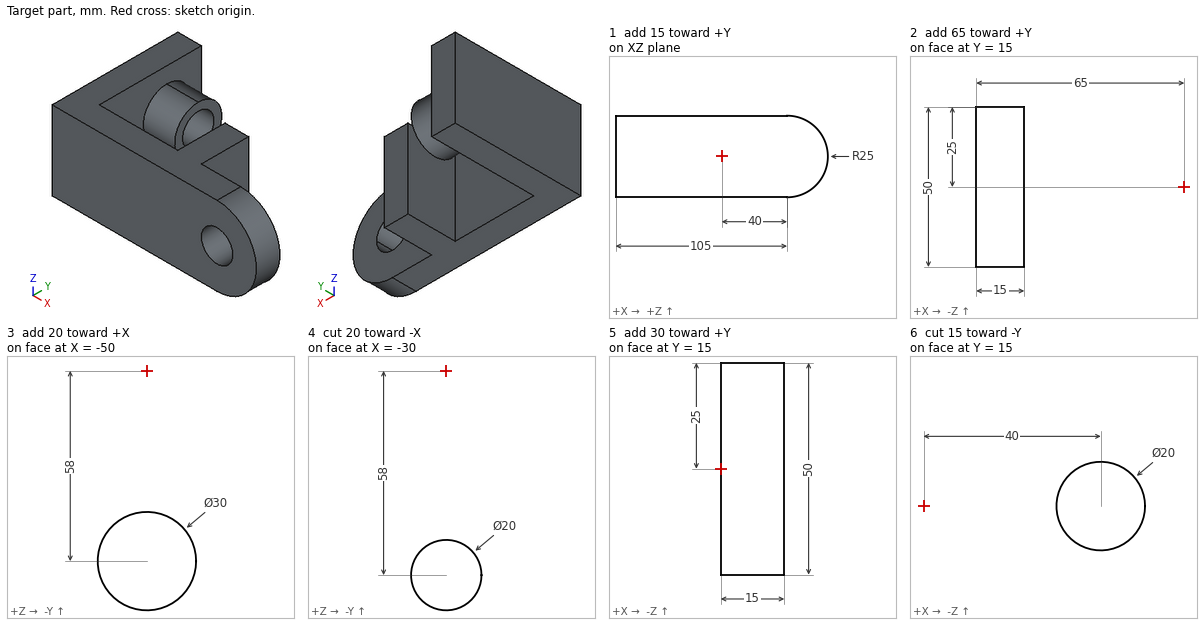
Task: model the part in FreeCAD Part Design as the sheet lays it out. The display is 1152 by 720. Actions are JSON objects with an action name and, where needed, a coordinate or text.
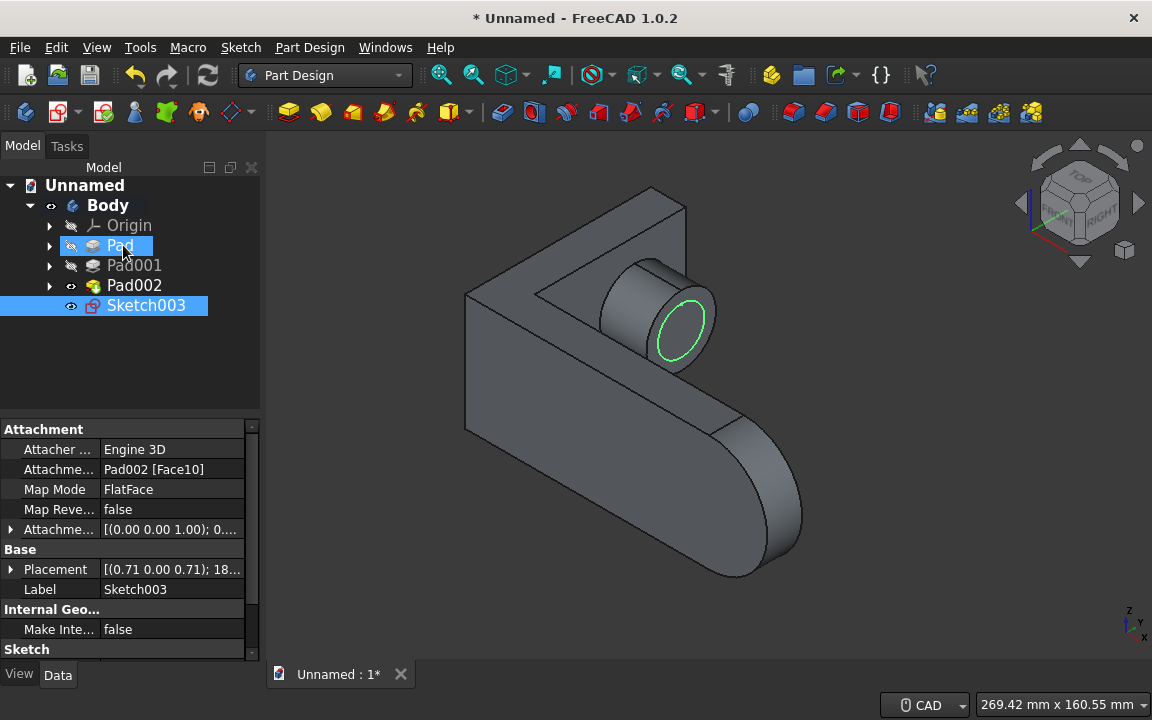
{"action": "left_click", "coordinate": [504, 112]}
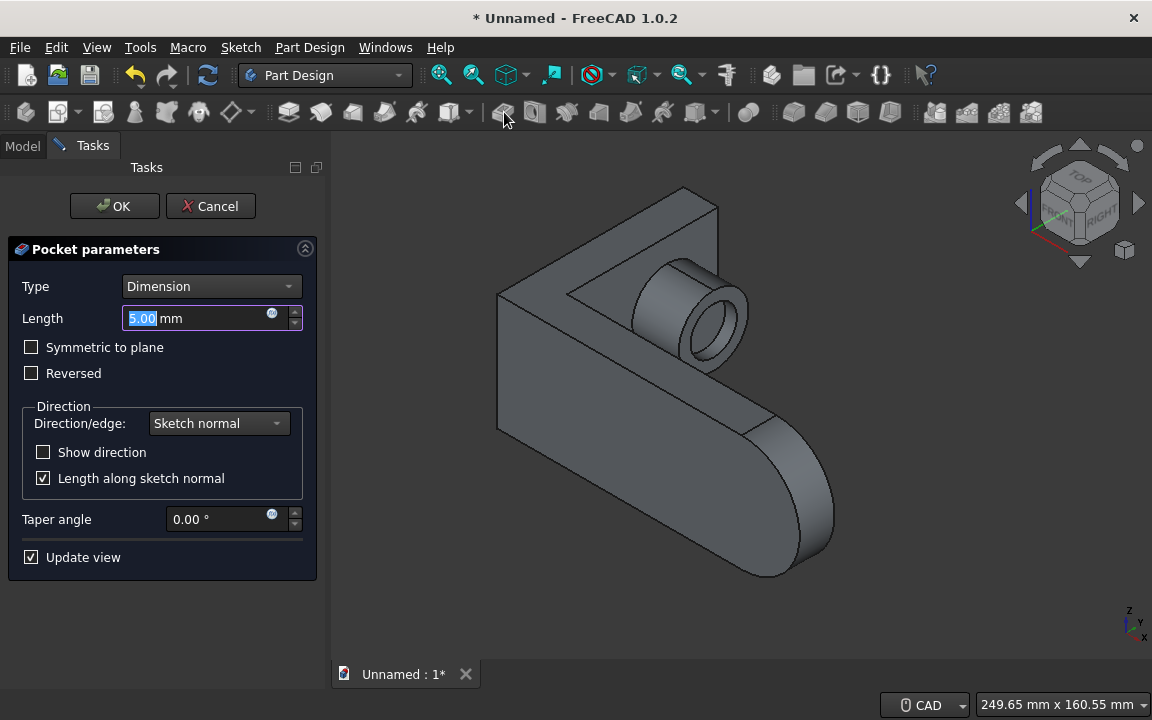
{"action": "type", "text": "20"}
{"action": "key", "text": "Tab"}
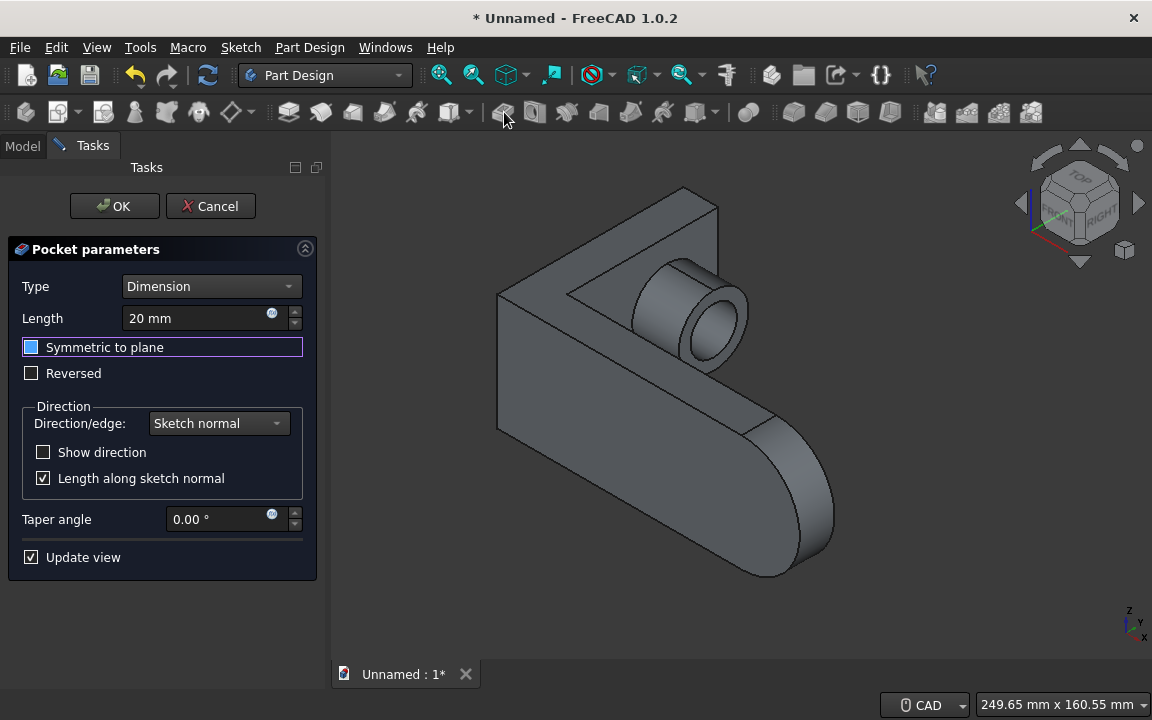
{"action": "left_click", "coordinate": [115, 206]}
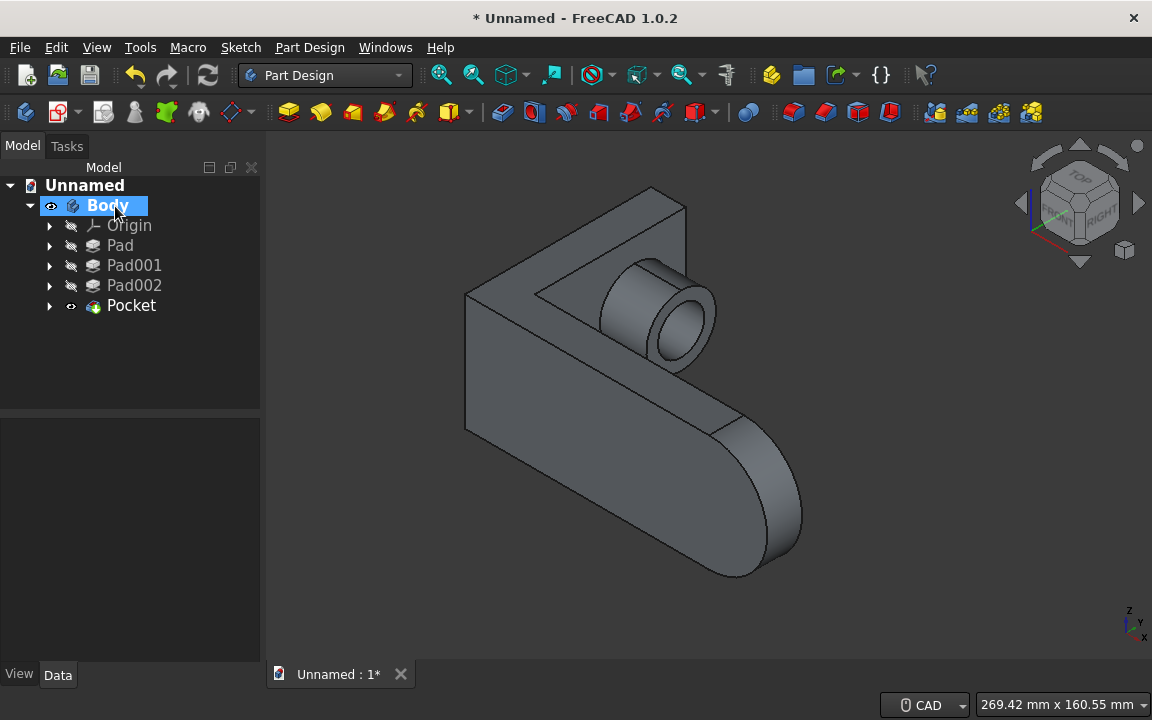
{"action": "key", "text": "4"}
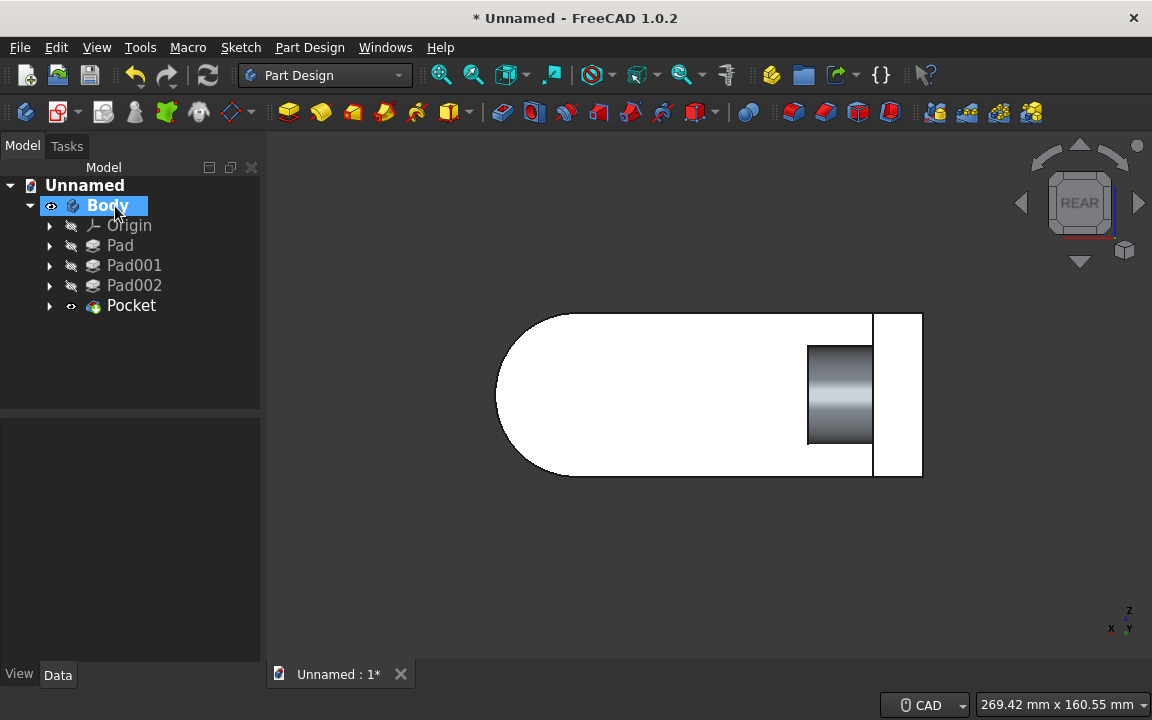
{"action": "left_click", "coordinate": [630, 394]}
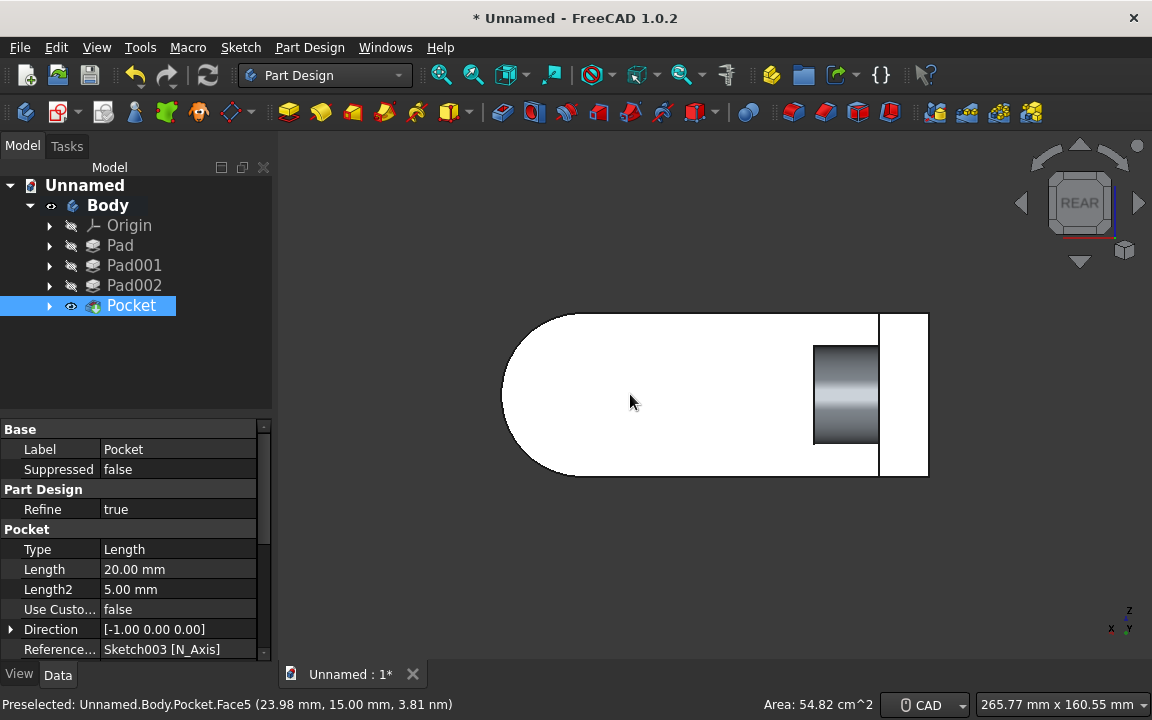
{"action": "left_click", "coordinate": [58, 112]}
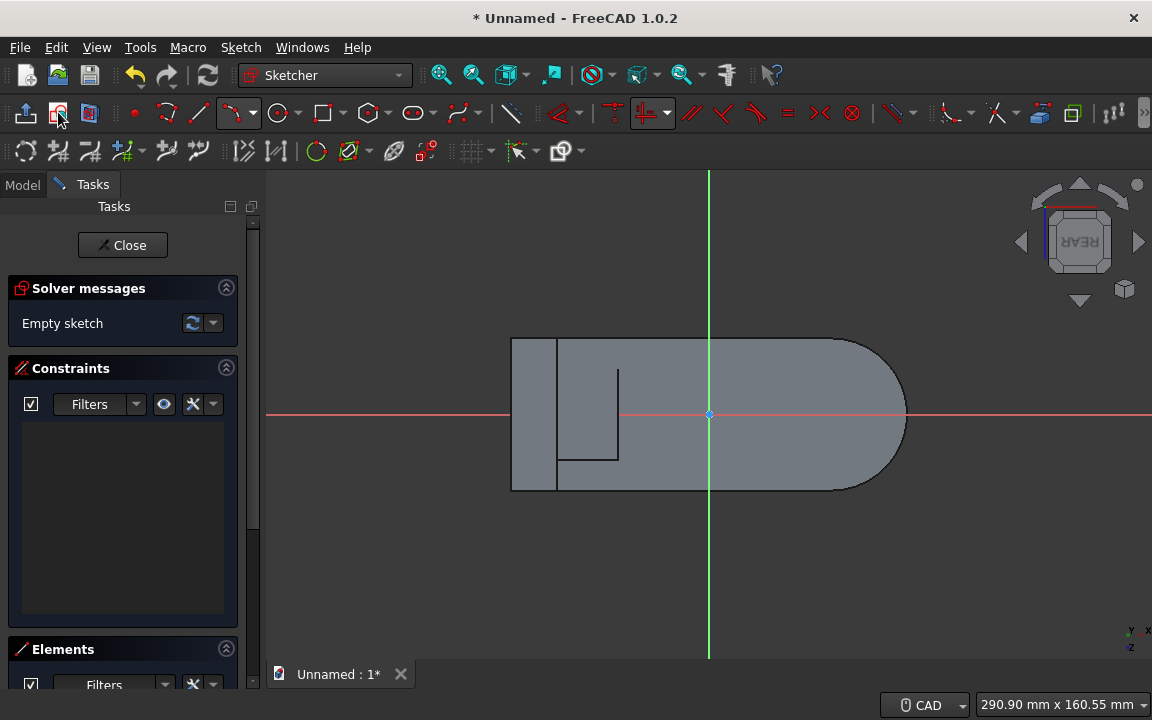
{"action": "scroll", "coordinate": [843, 415], "scroll_direction": "up", "scroll_amount": 3}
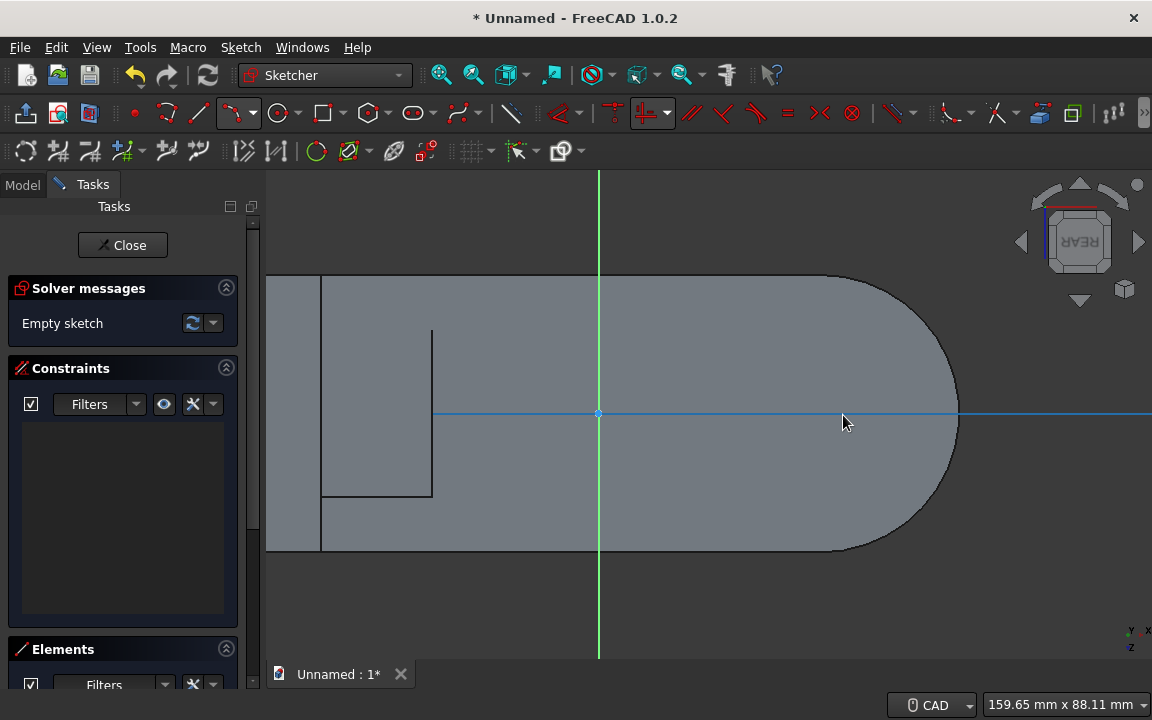
{"action": "left_click", "coordinate": [324, 114]}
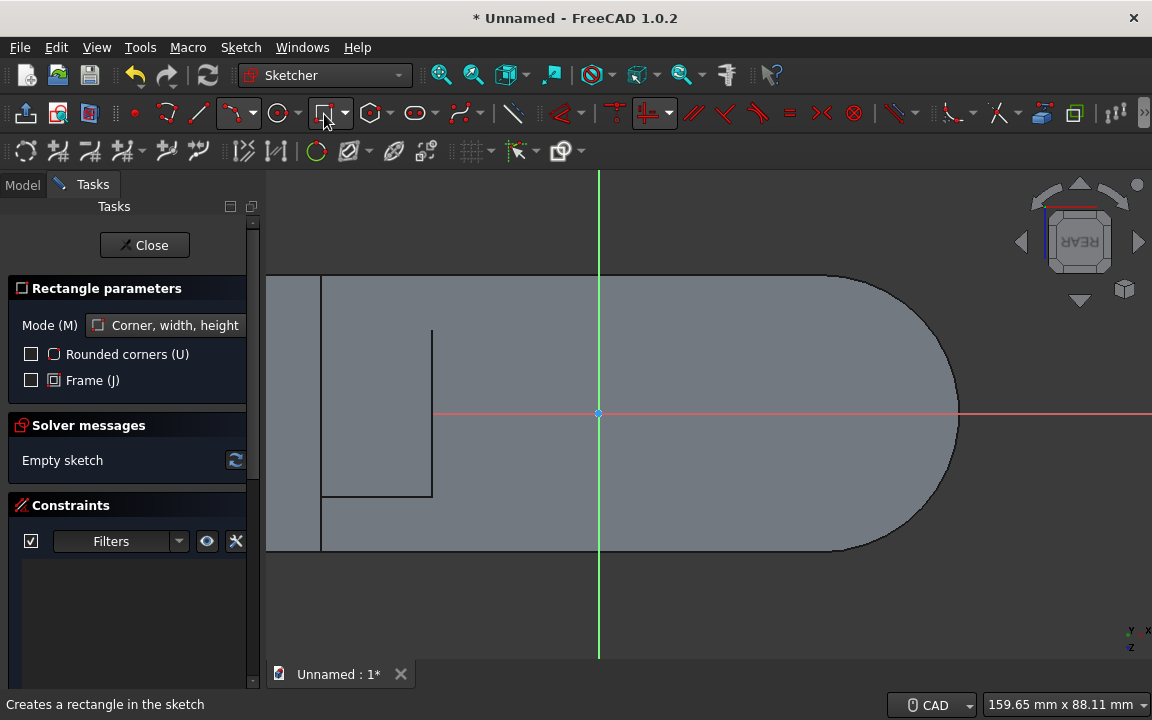
{"action": "left_click", "coordinate": [599, 275]}
{"action": "mouse_move", "coordinate": [682, 552]}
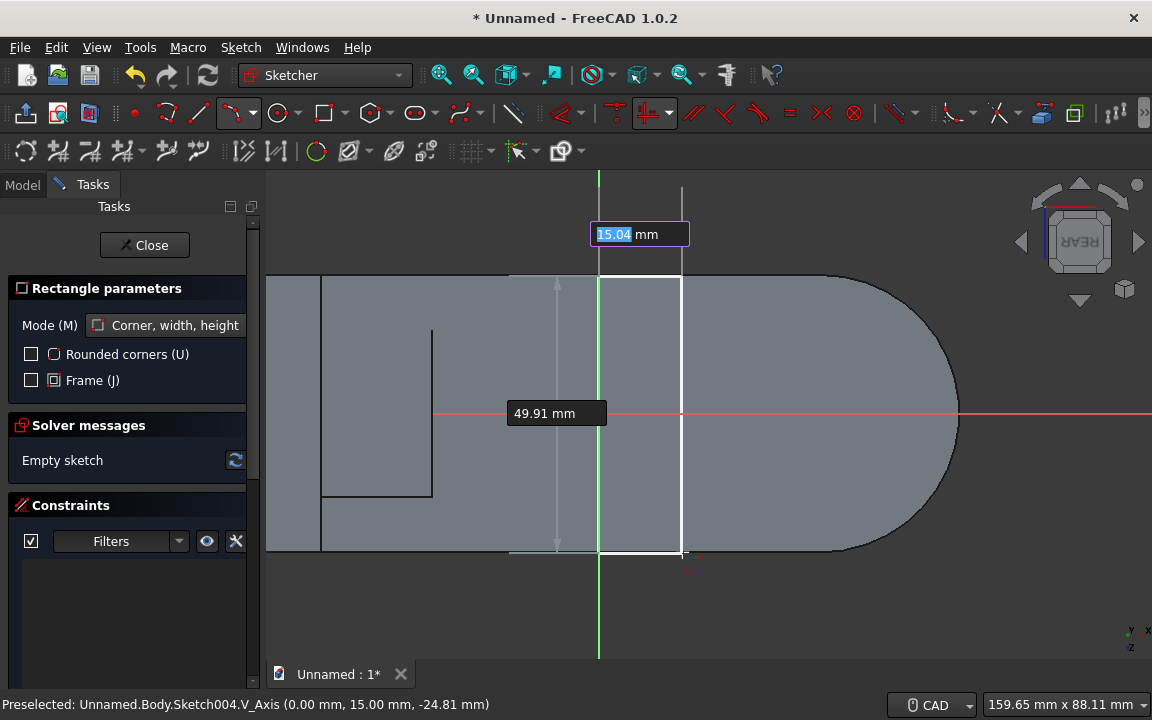
{"action": "type", "text": "15"}
{"action": "key", "text": "Tab"}
{"action": "type", "text": "50"}
{"action": "key", "text": "Return"}
{"action": "key", "text": "Escape"}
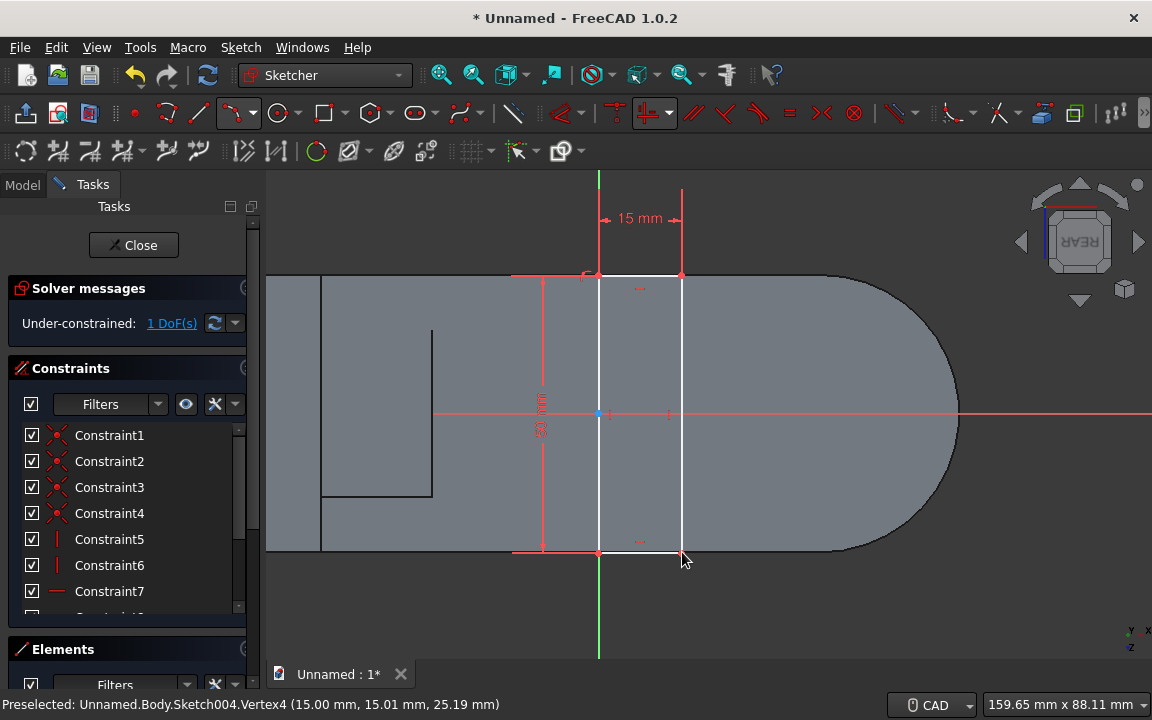
{"action": "left_click", "coordinate": [560, 114]}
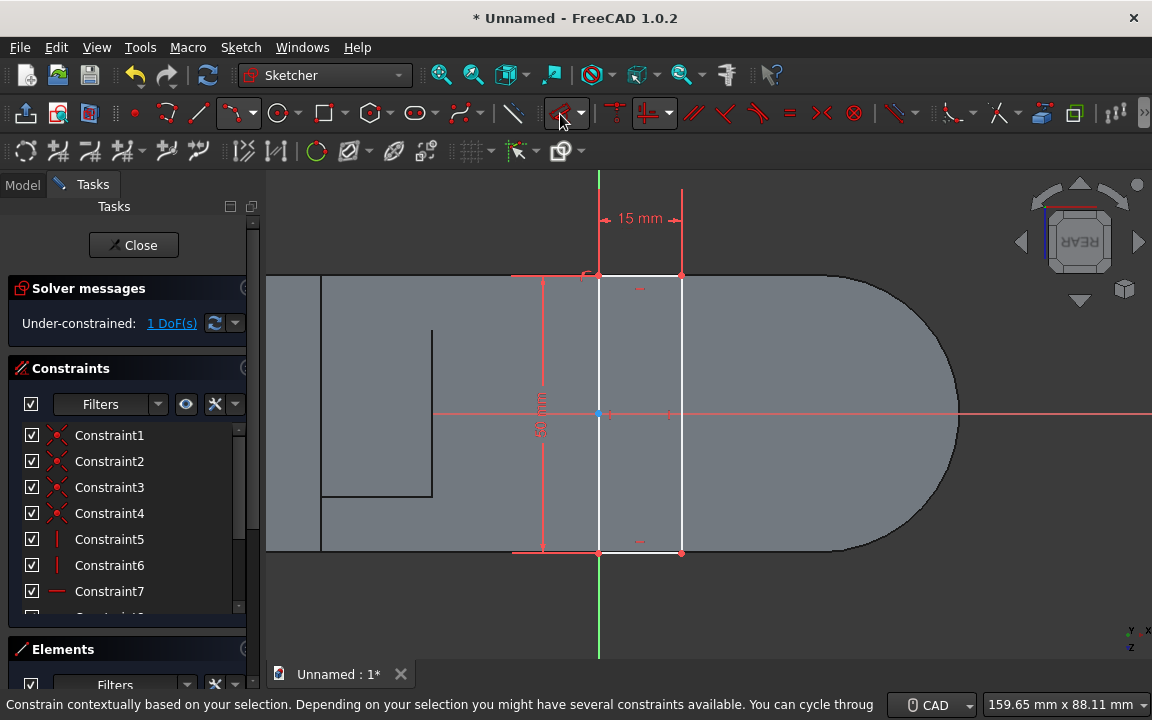
{"action": "left_click", "coordinate": [599, 276]}
{"action": "left_click", "coordinate": [565, 345]}